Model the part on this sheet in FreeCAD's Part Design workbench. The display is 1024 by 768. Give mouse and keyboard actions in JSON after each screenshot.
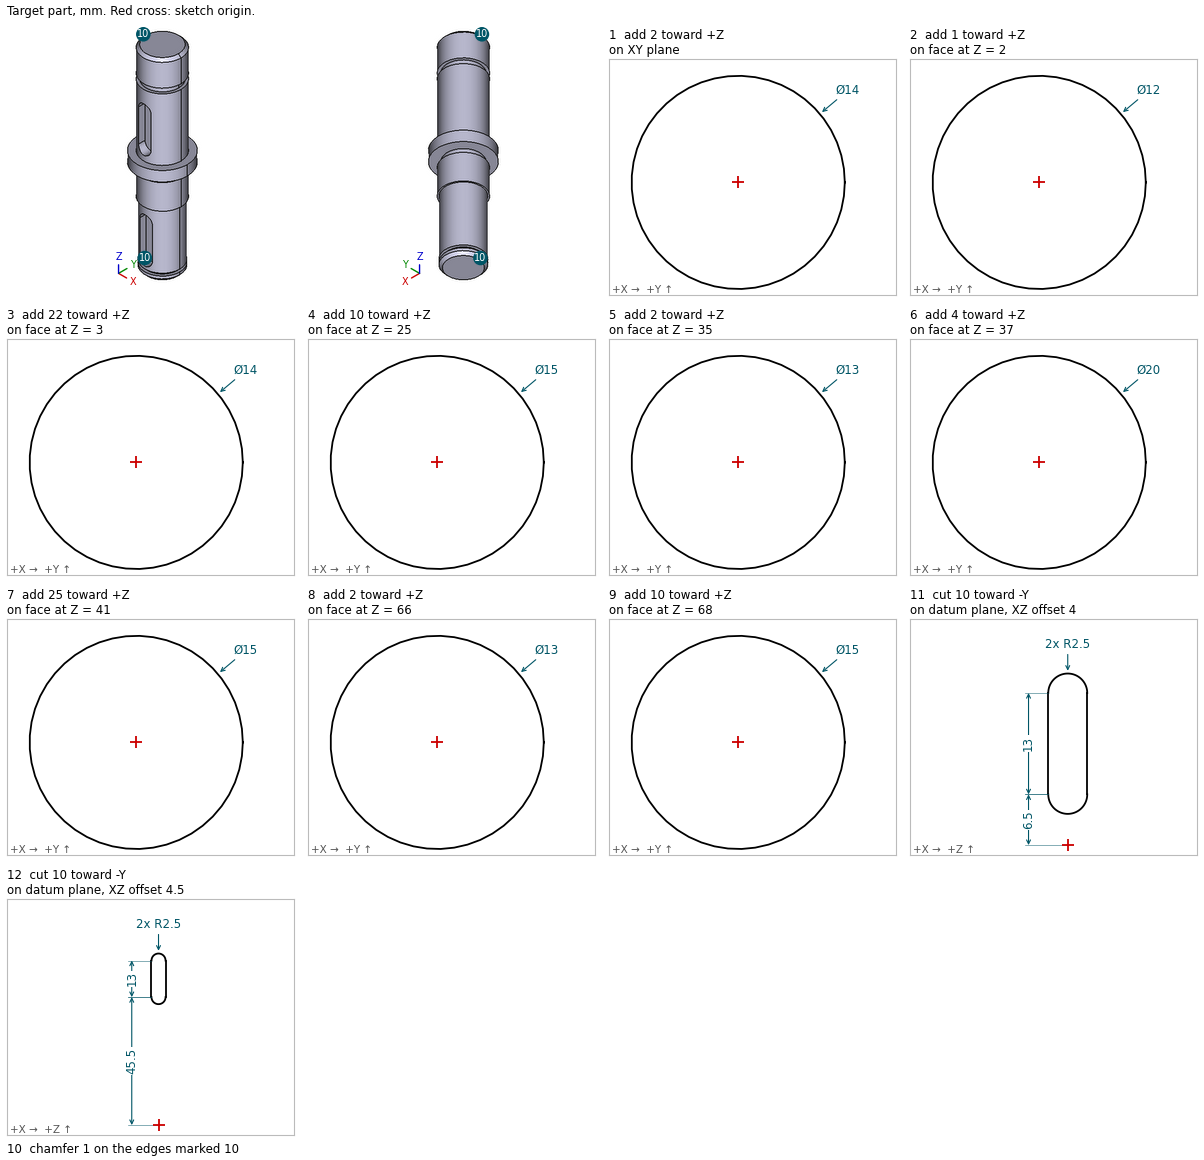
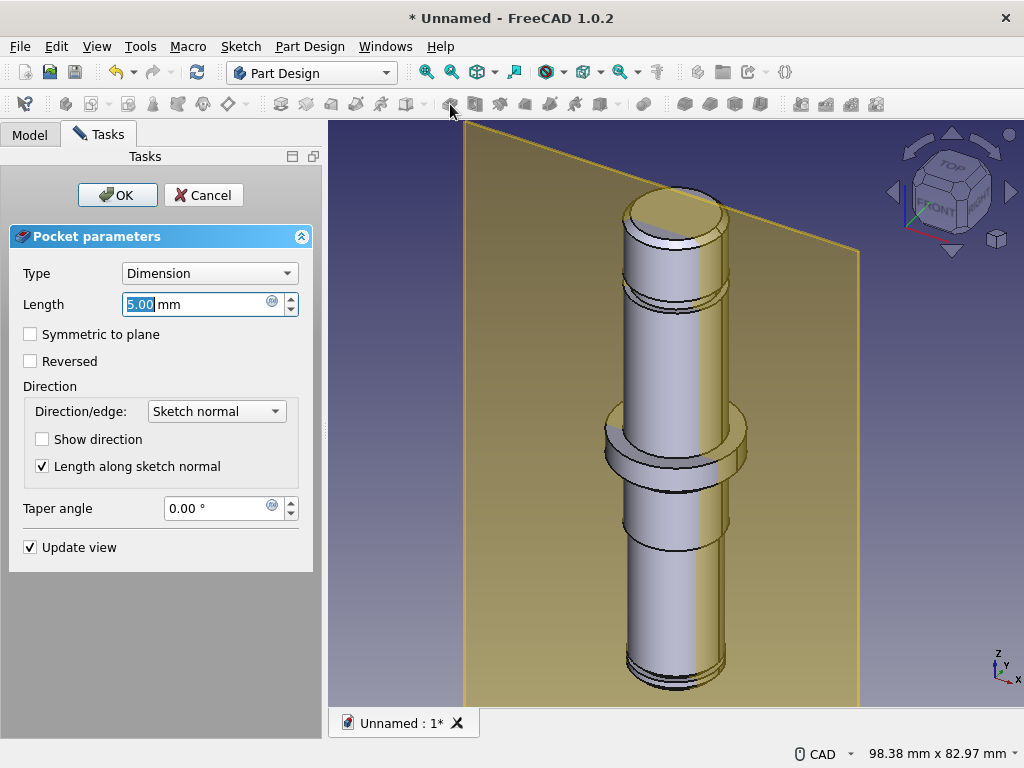
{"action": "type", "text": "10"}
{"action": "key", "text": "Tab"}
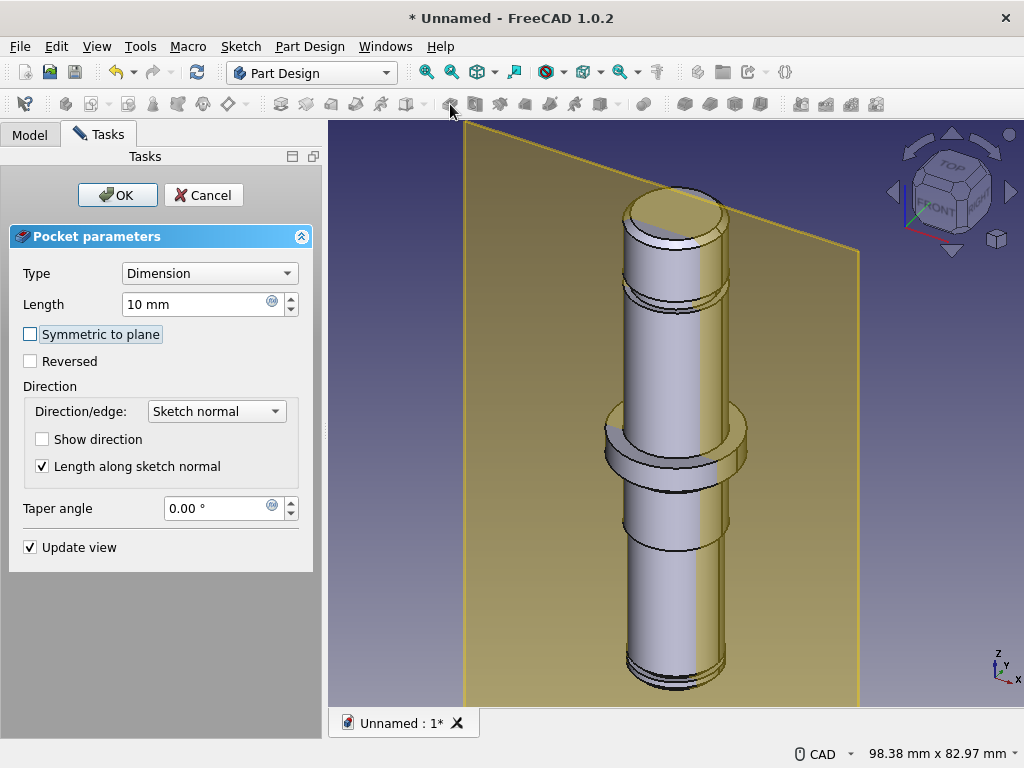
{"action": "left_click", "coordinate": [31, 361]}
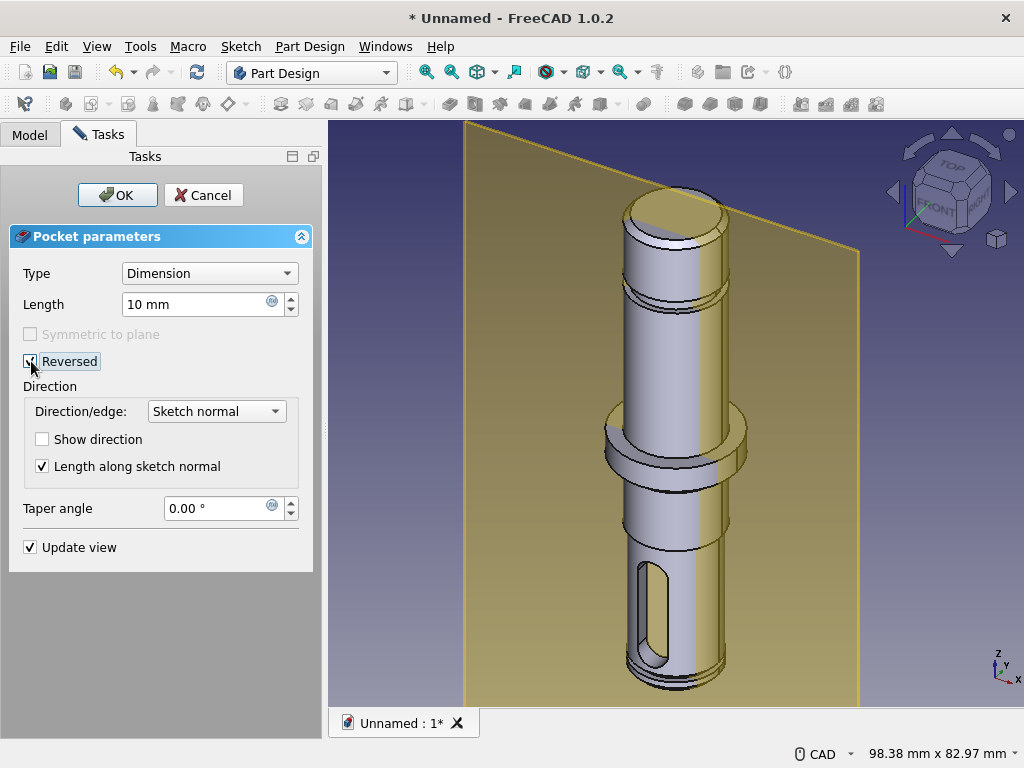
{"action": "left_click", "coordinate": [118, 195]}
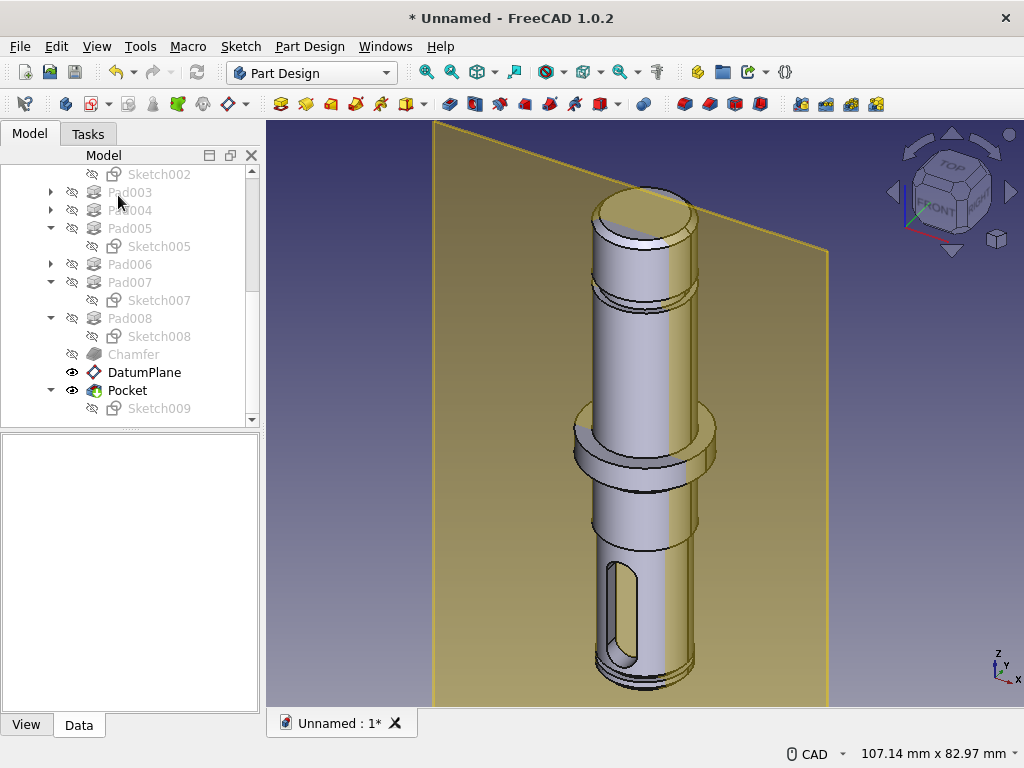
{"action": "left_click", "coordinate": [117, 372]}
{"action": "key", "text": "space"}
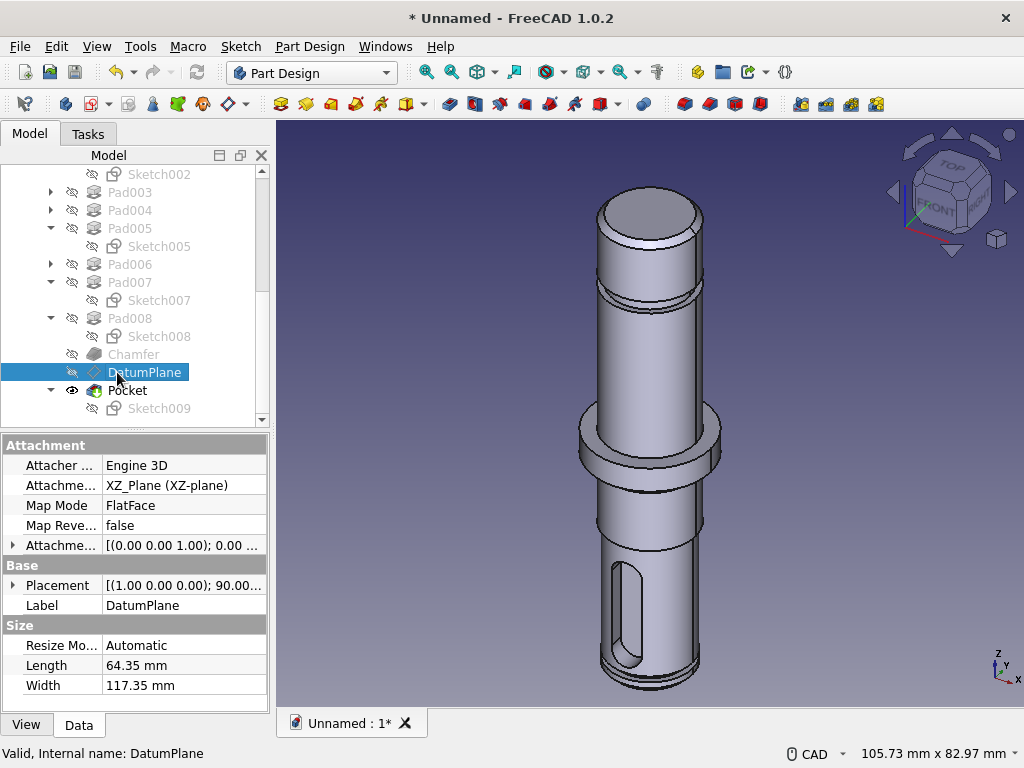
{"action": "left_click", "coordinate": [427, 72]}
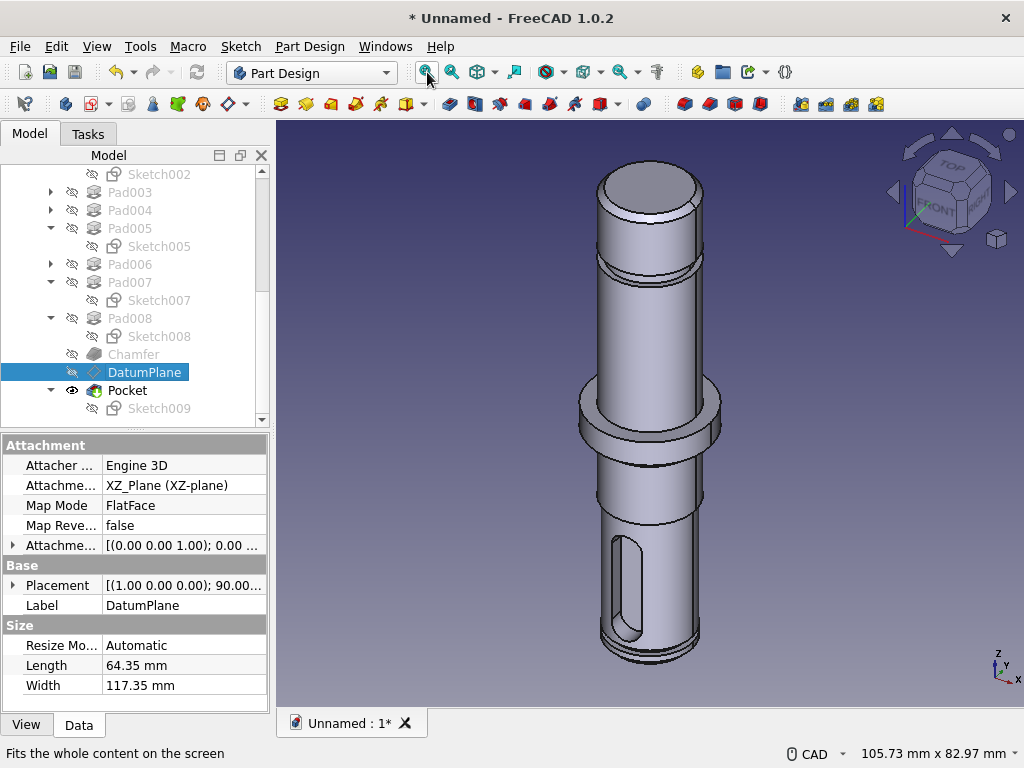
{"action": "scroll", "coordinate": [161, 296], "scroll_direction": "down", "scroll_amount": 3}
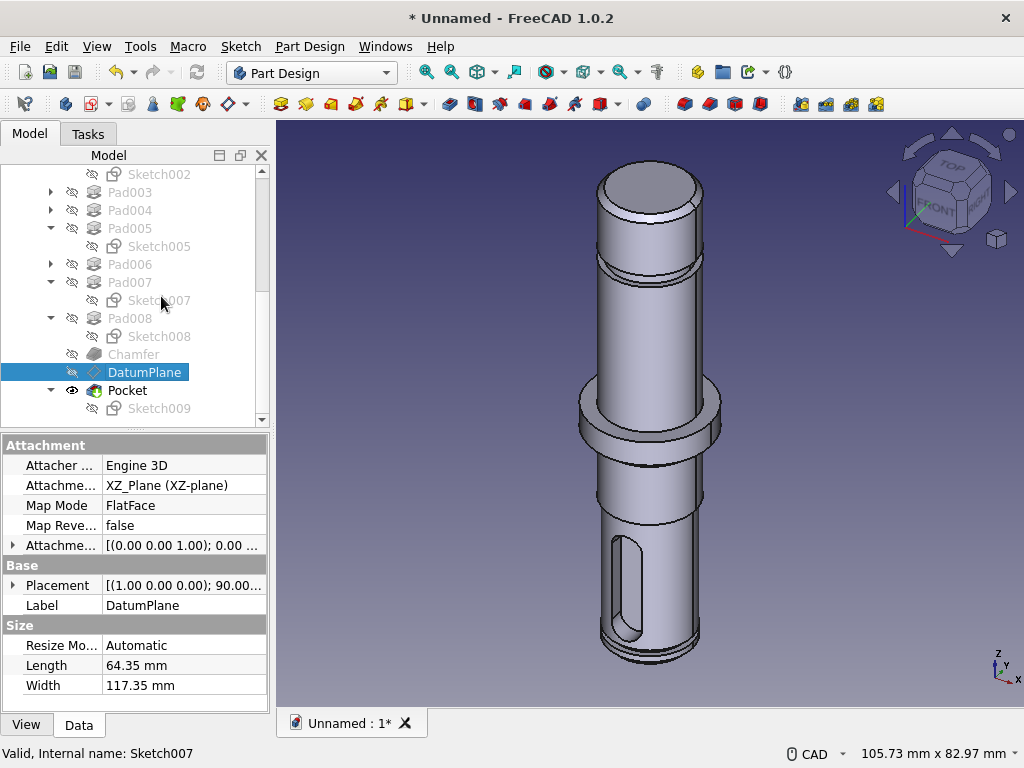
{"action": "scroll", "coordinate": [161, 296], "scroll_direction": "up", "scroll_amount": 15}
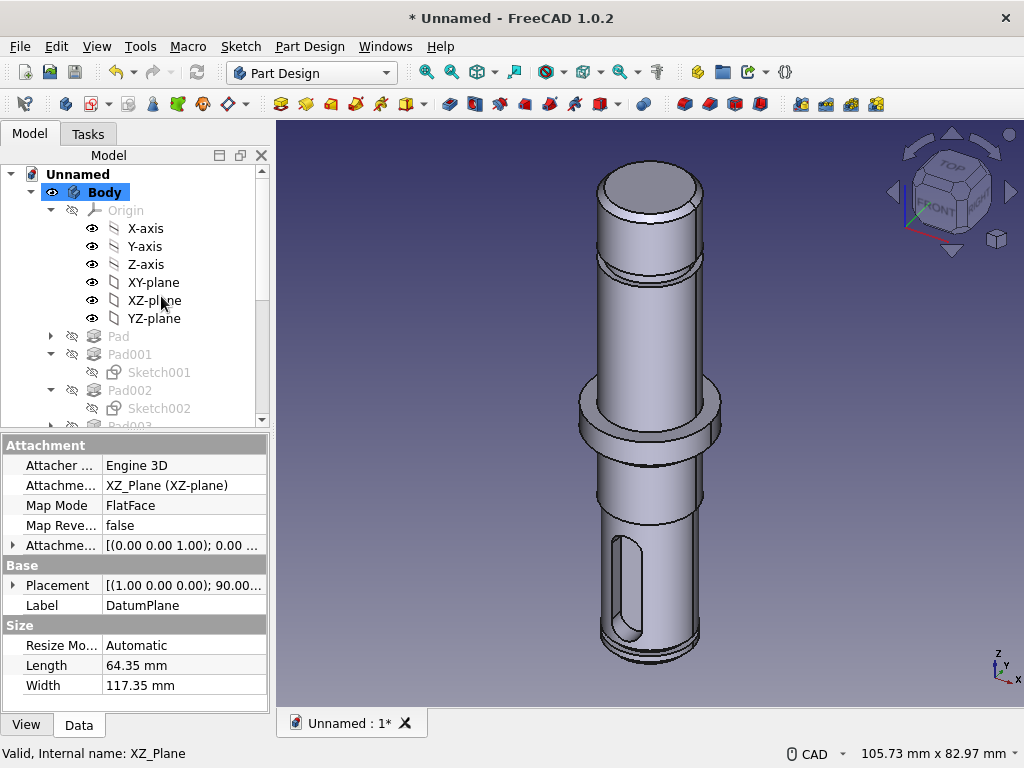
{"action": "left_click", "coordinate": [137, 300]}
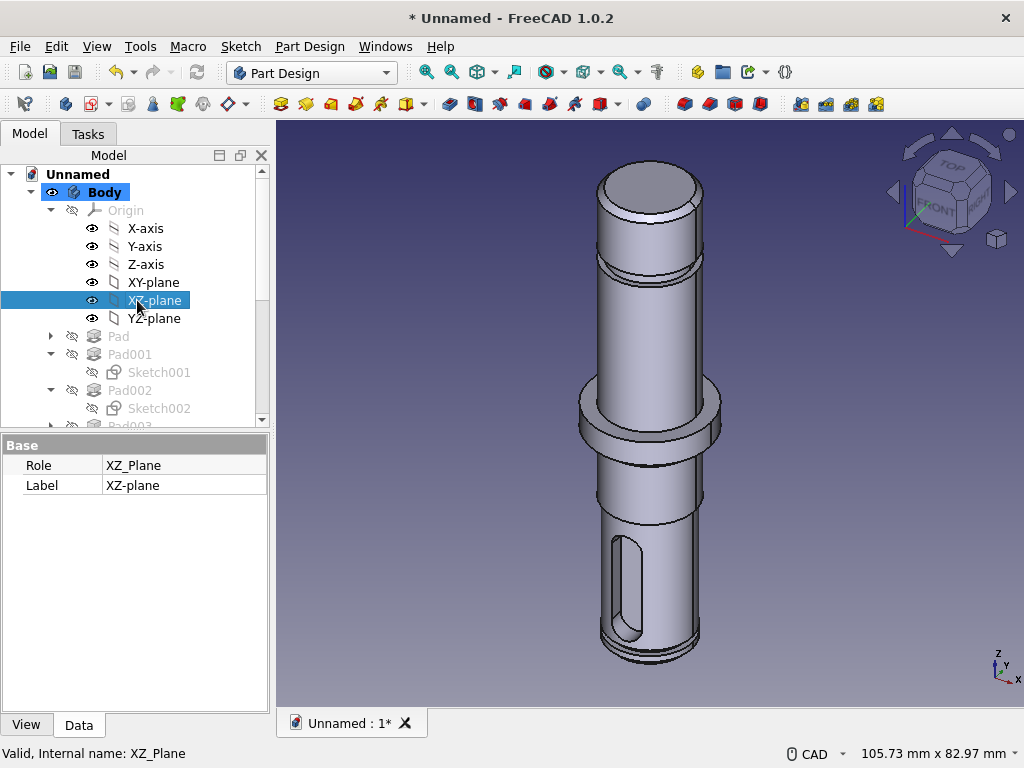
{"action": "left_click", "coordinate": [228, 104]}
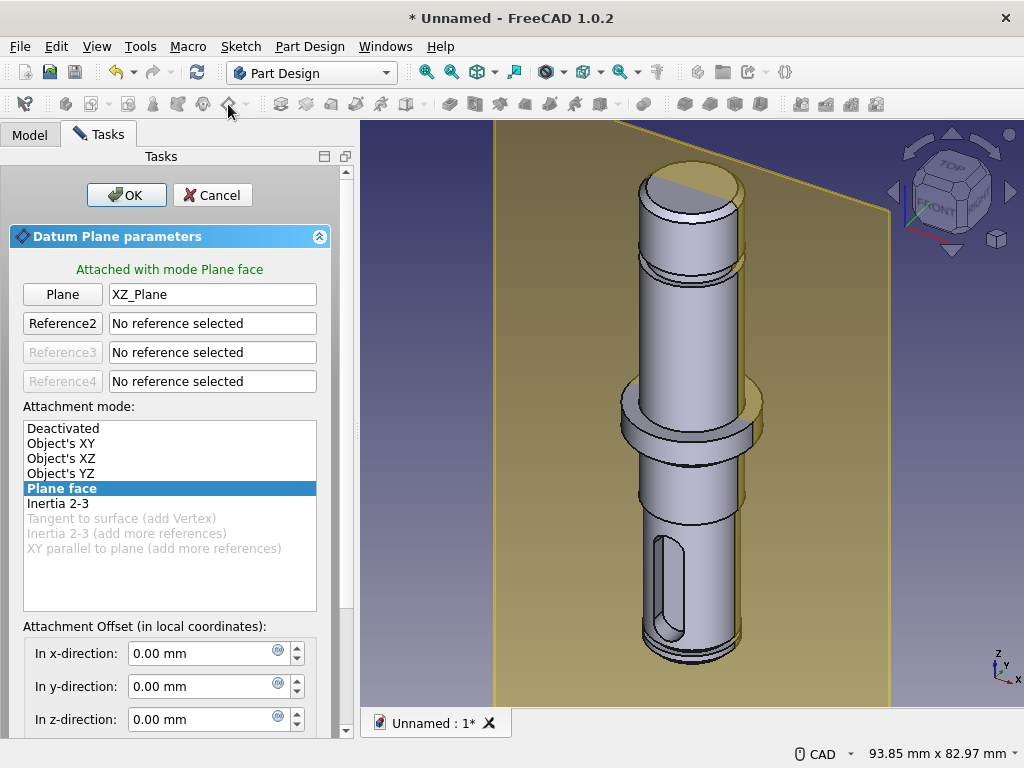
{"action": "triple_click", "coordinate": [210, 720]}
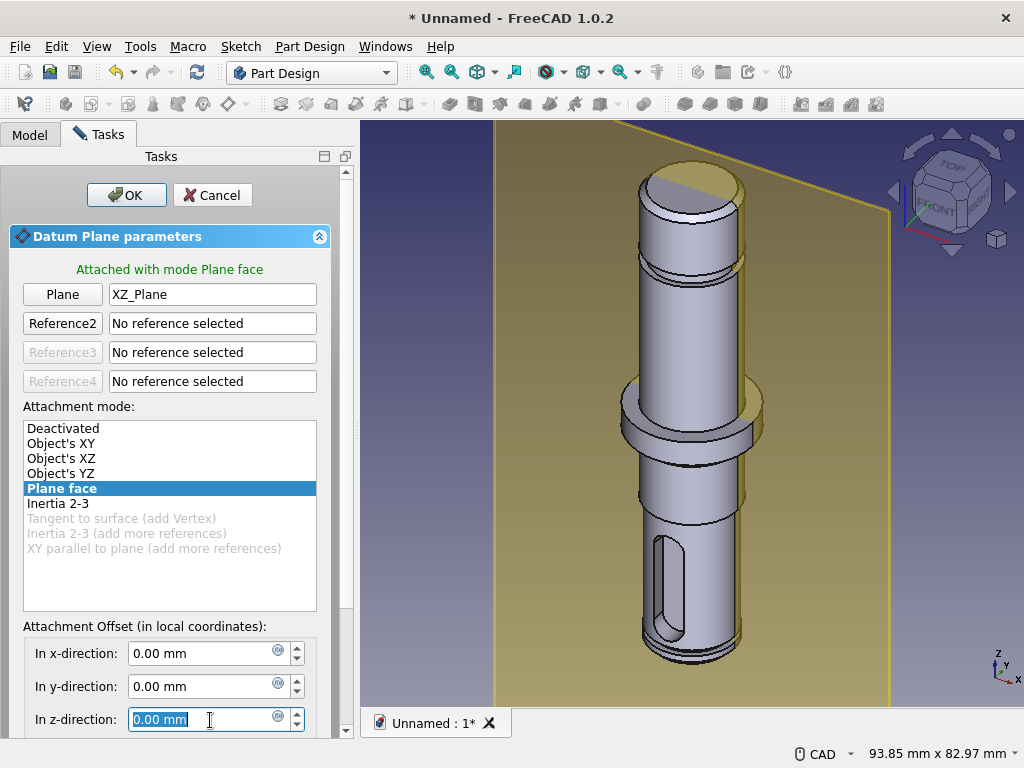
{"action": "type", "text": "4.5"}
{"action": "key", "text": "Tab"}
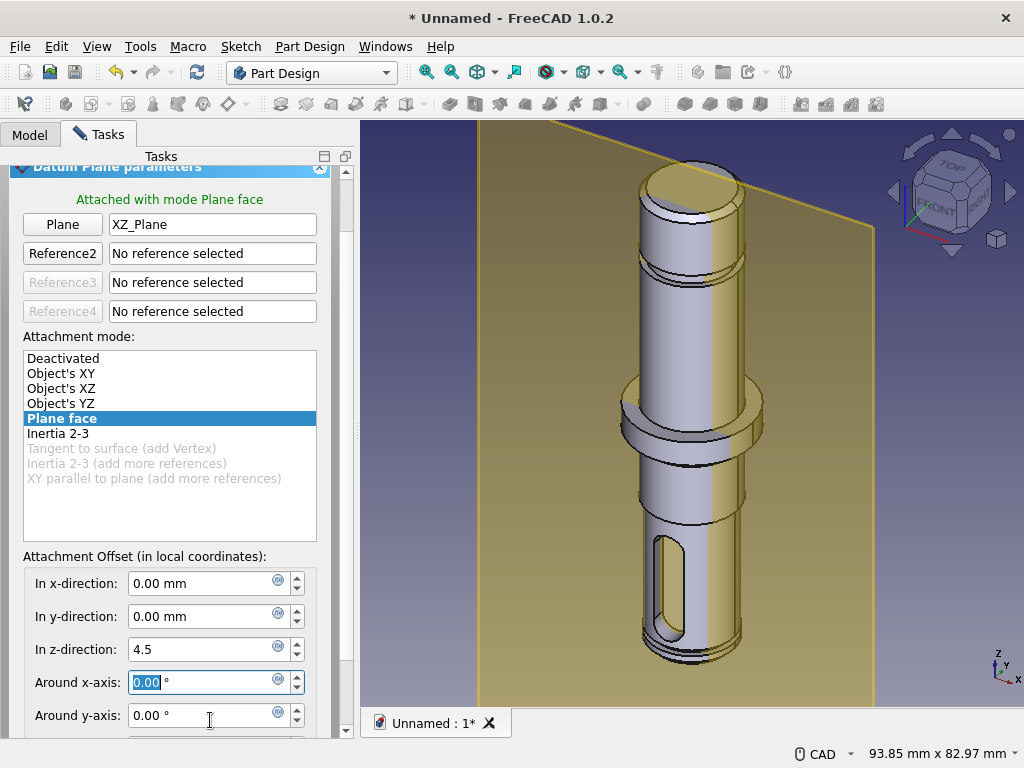
{"action": "scroll", "coordinate": [346, 452], "scroll_direction": "up", "scroll_amount": 2}